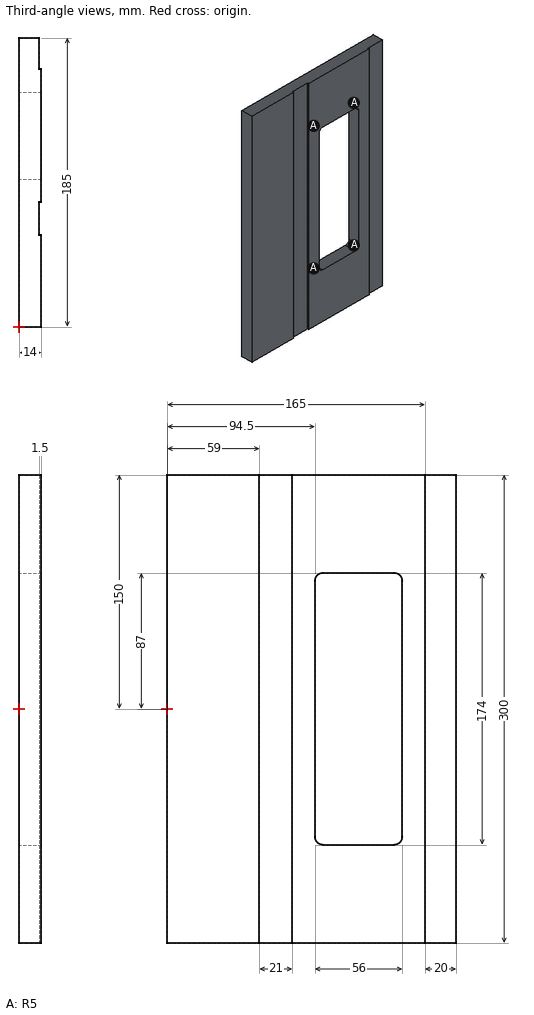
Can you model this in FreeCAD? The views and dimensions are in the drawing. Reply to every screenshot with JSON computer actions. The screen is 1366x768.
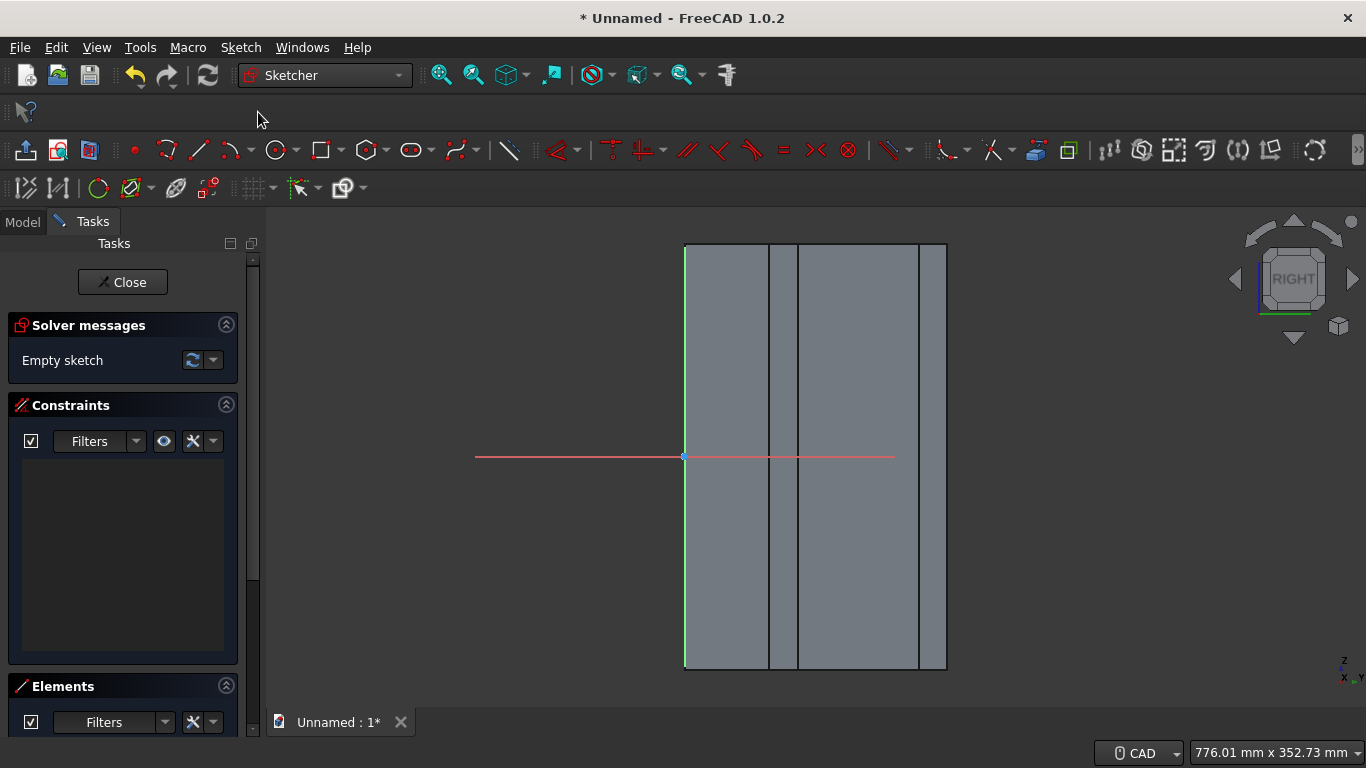
{"action": "left_click", "coordinate": [322, 150]}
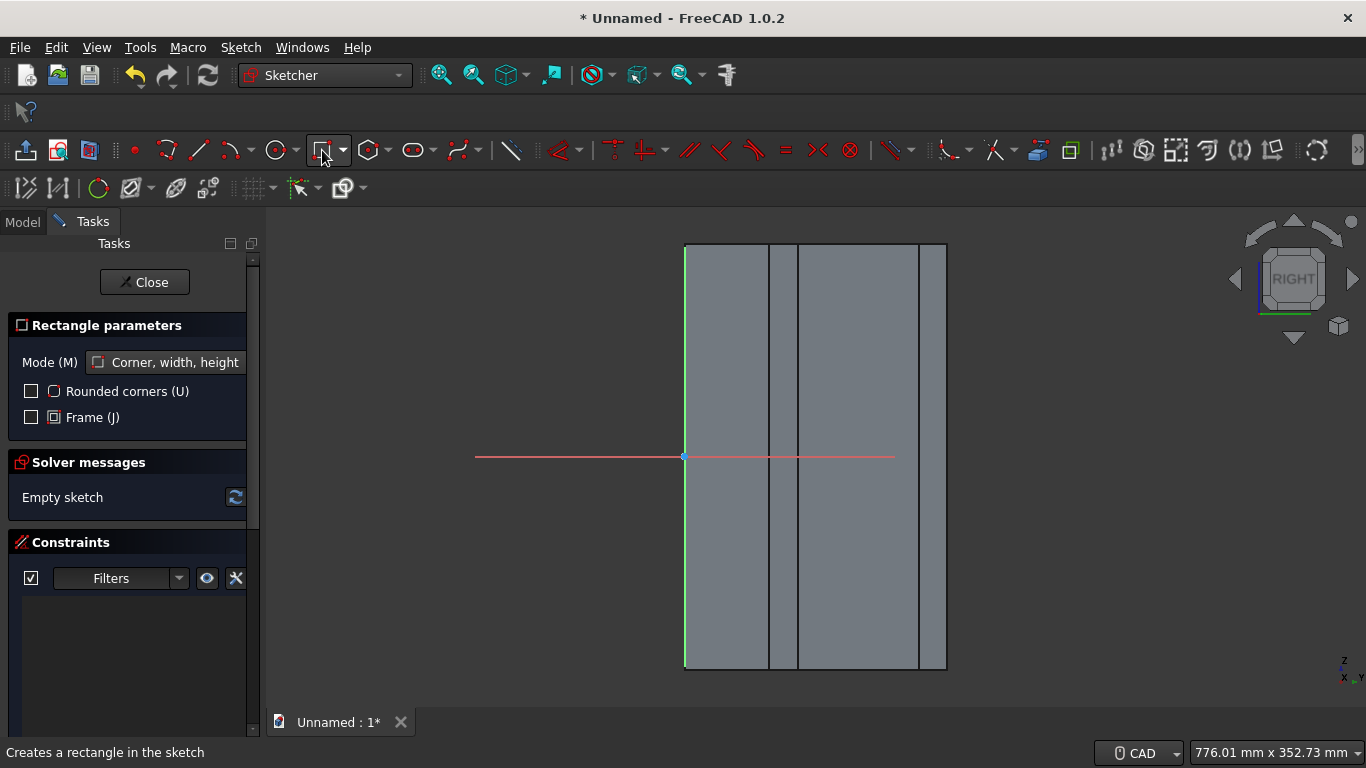
{"action": "left_click", "coordinate": [819, 334]}
{"action": "left_click", "coordinate": [898, 580]}
{"action": "key", "text": "Escape"}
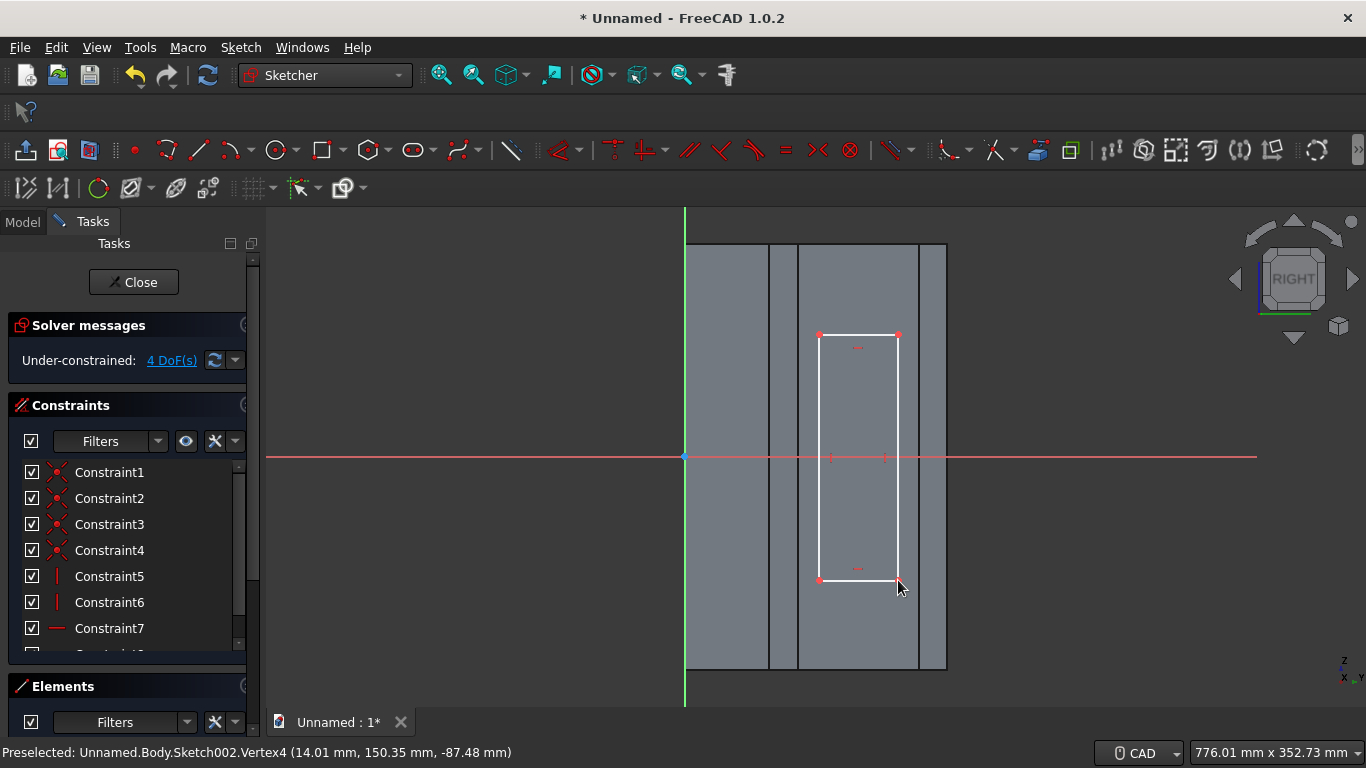
{"action": "key", "text": "d"}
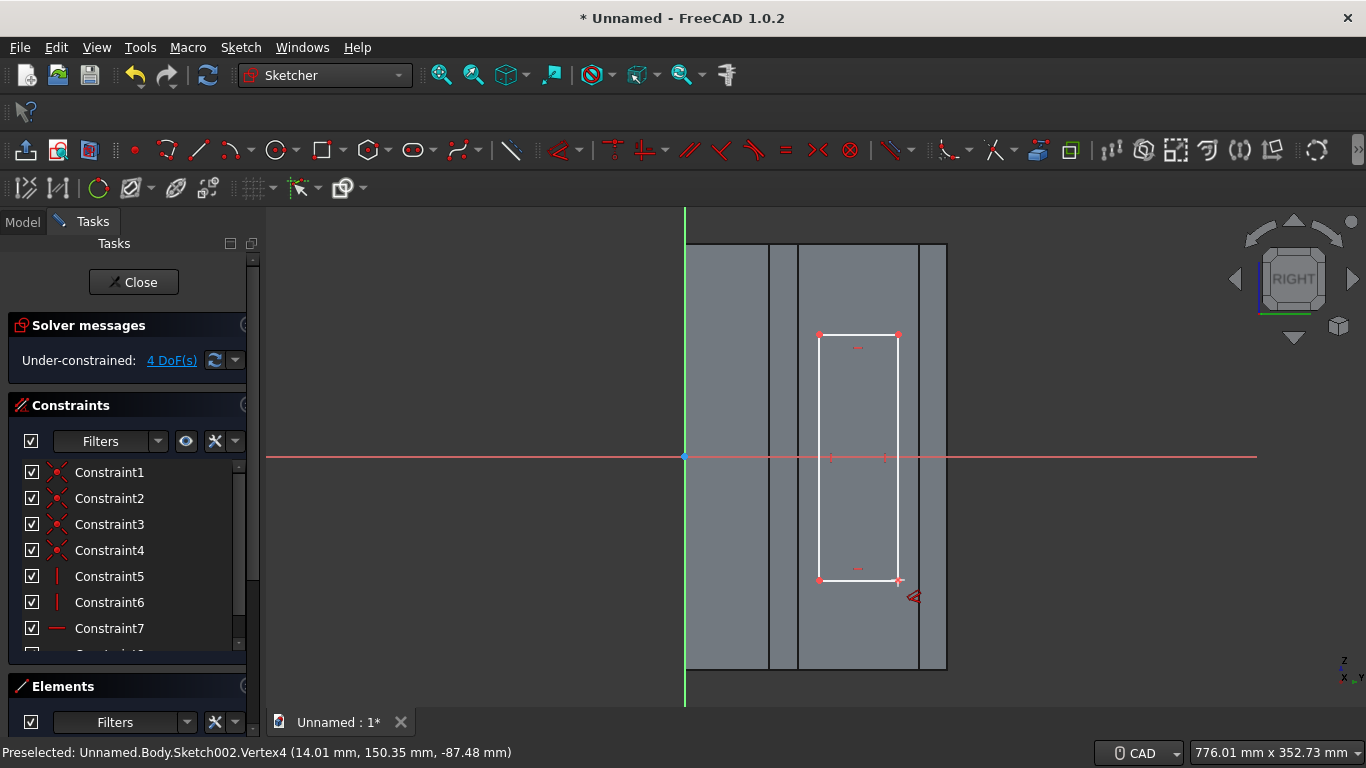
{"action": "left_click", "coordinate": [843, 581]}
{"action": "left_click", "coordinate": [858, 615]}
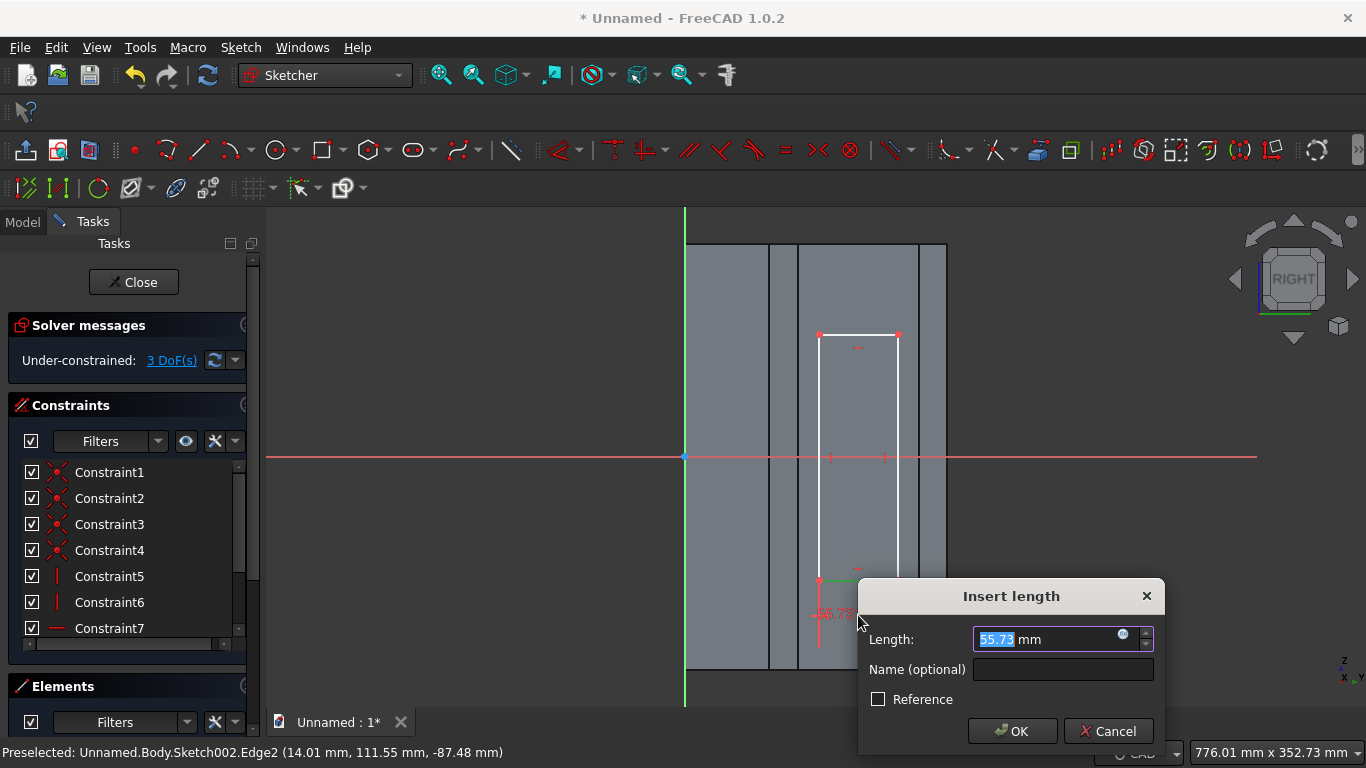
{"action": "type", "text": "56"}
{"action": "key", "text": "Return"}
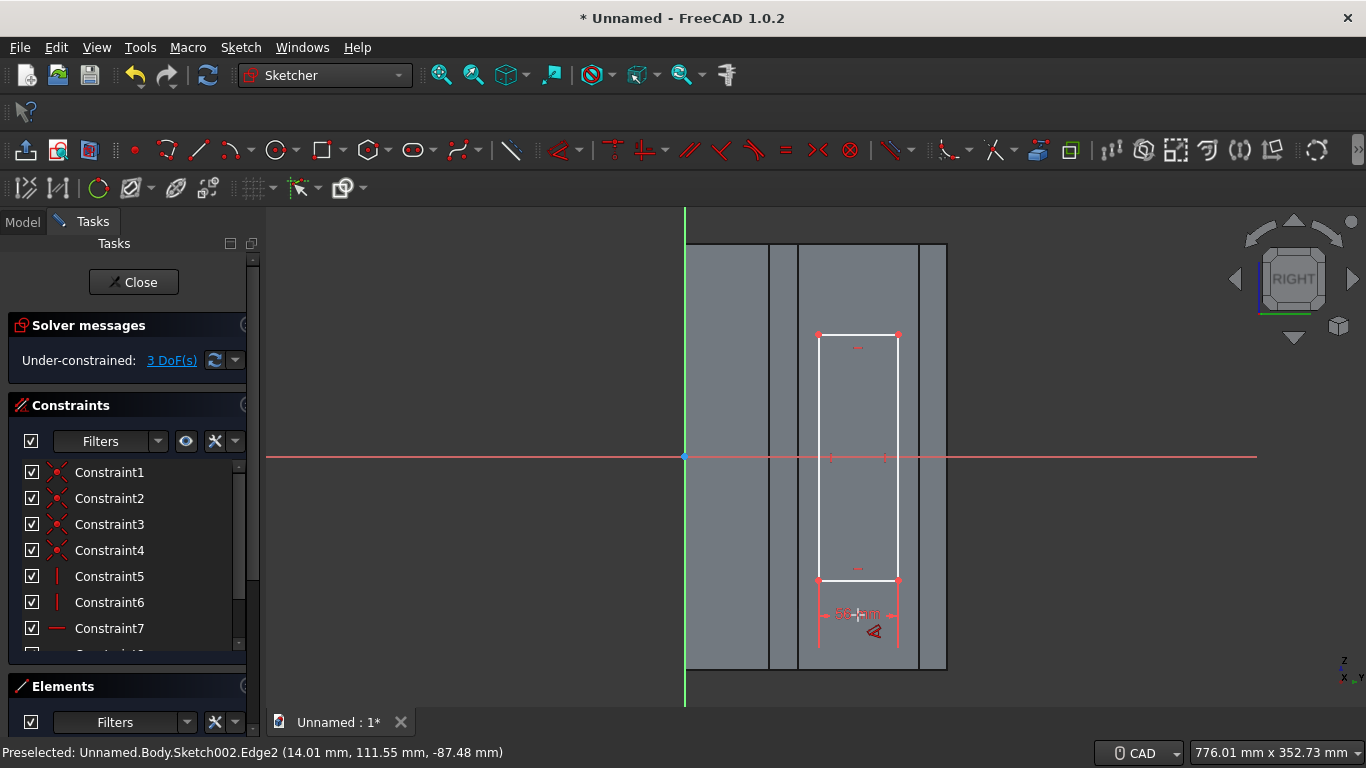
{"action": "left_click", "coordinate": [819, 409]}
{"action": "left_click", "coordinate": [853, 401]}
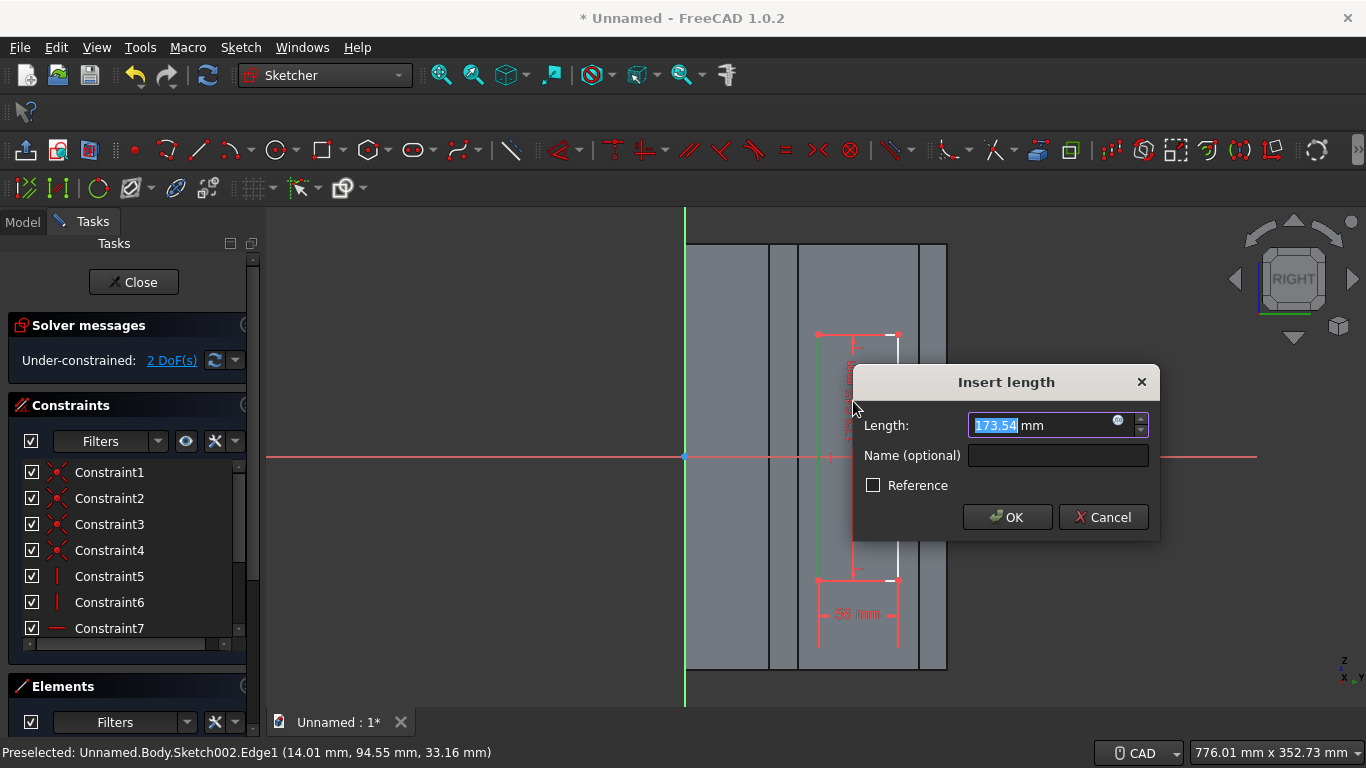
{"action": "type", "text": "174"}
{"action": "key", "text": "Return"}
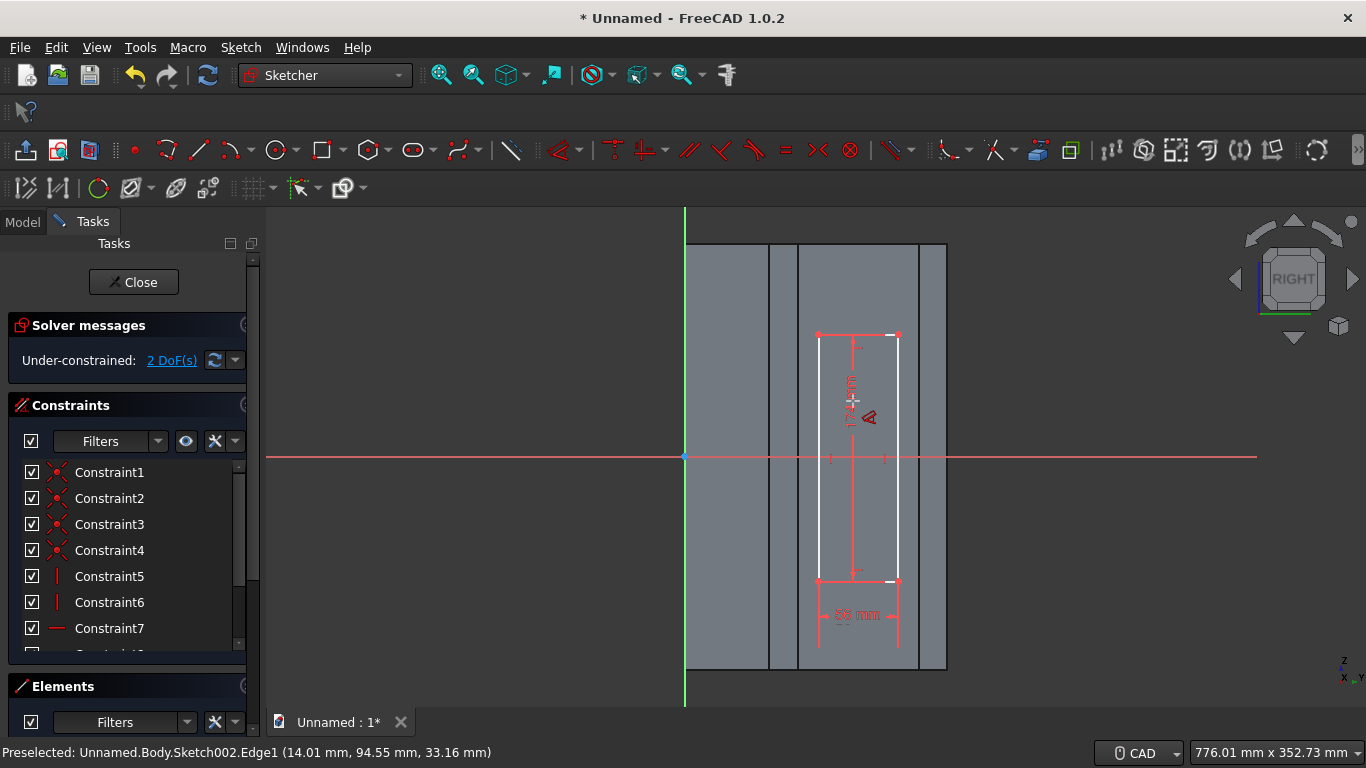
{"action": "left_click", "coordinate": [819, 335]}
{"action": "left_click", "coordinate": [651, 396]}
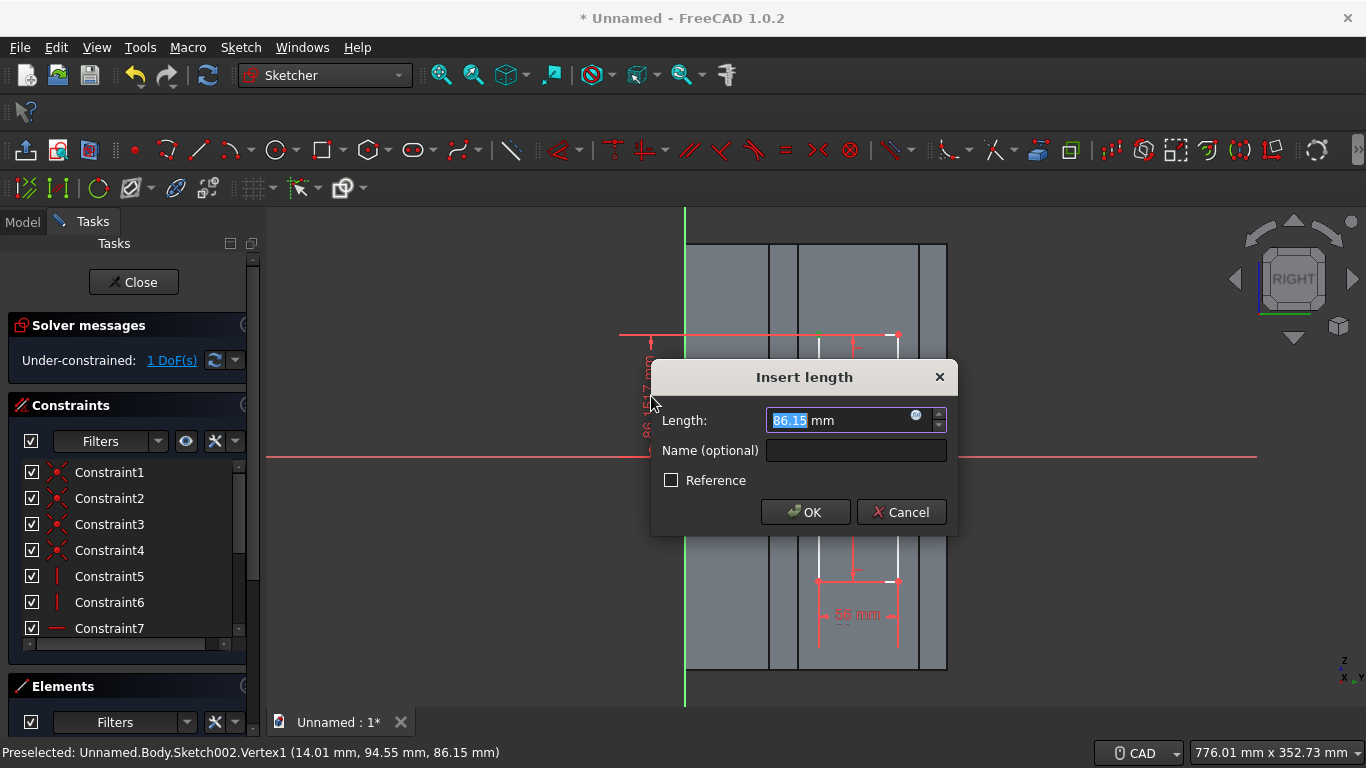
{"action": "type", "text": "87"}
{"action": "key", "text": "Return"}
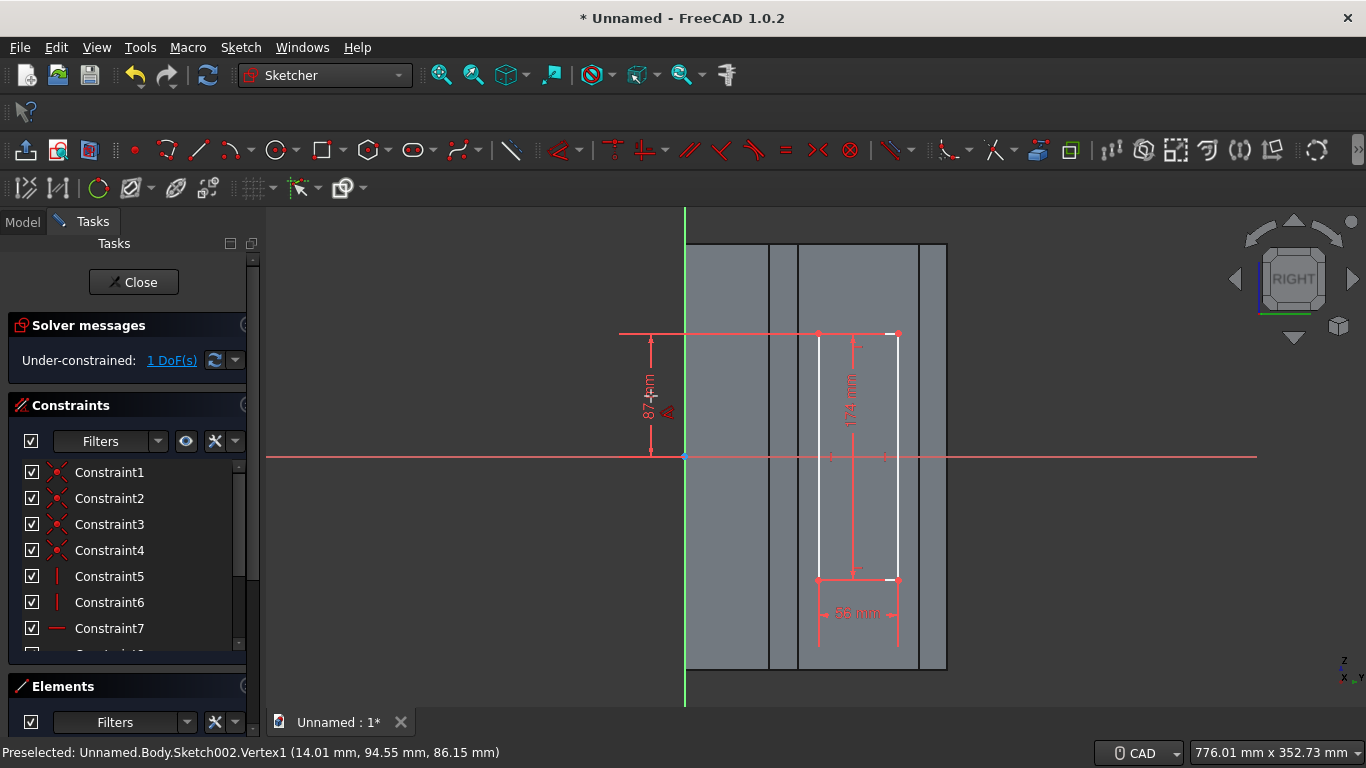
{"action": "left_click", "coordinate": [819, 334]}
{"action": "left_click", "coordinate": [752, 300]}